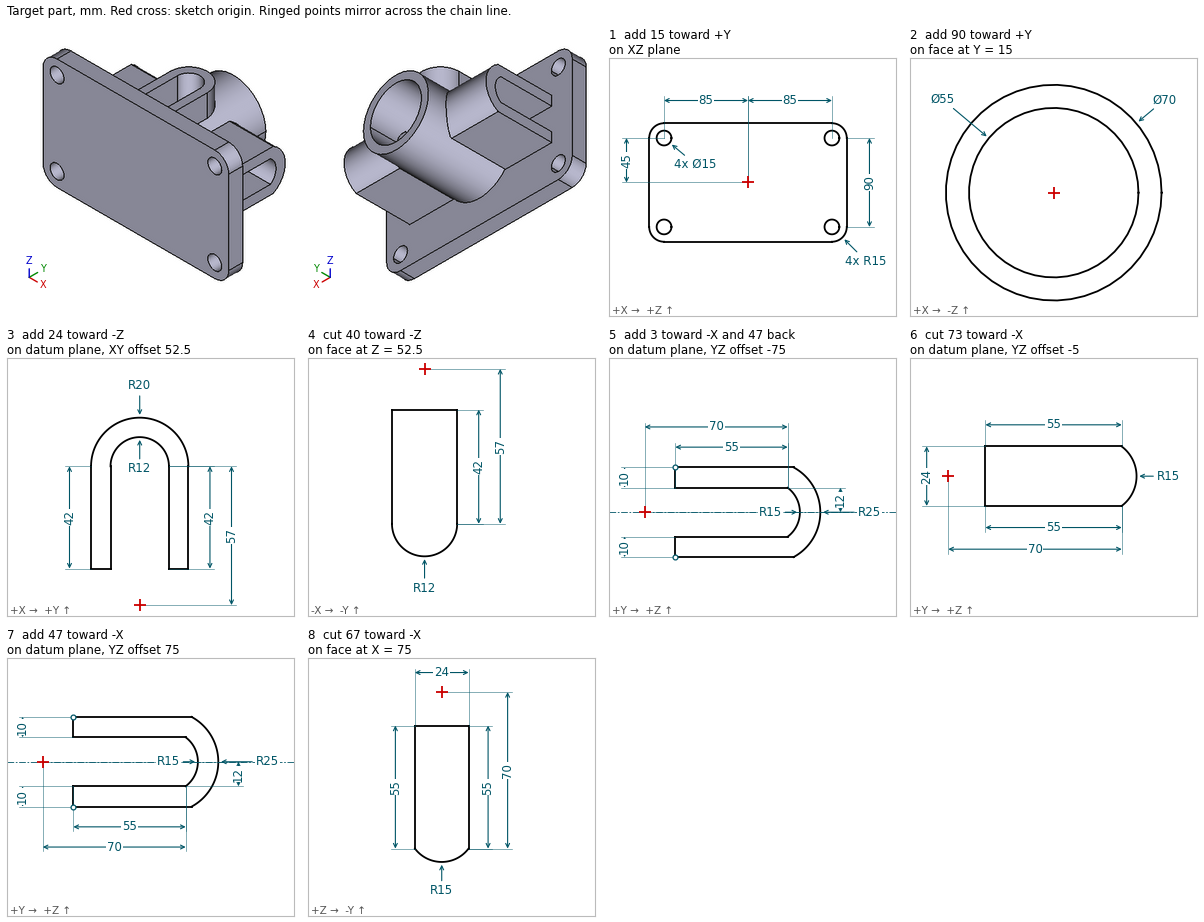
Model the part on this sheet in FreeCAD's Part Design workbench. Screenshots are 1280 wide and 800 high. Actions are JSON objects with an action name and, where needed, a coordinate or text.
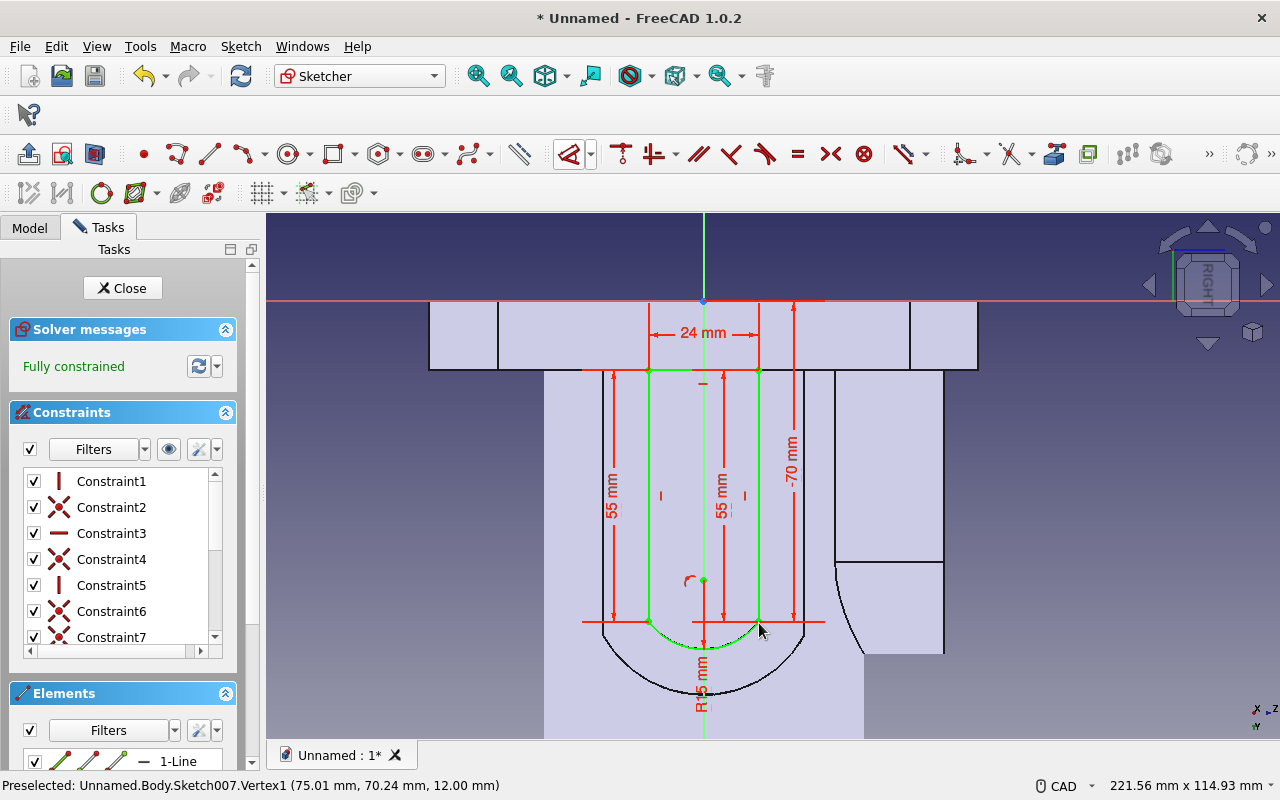
{"action": "left_click", "coordinate": [123, 288]}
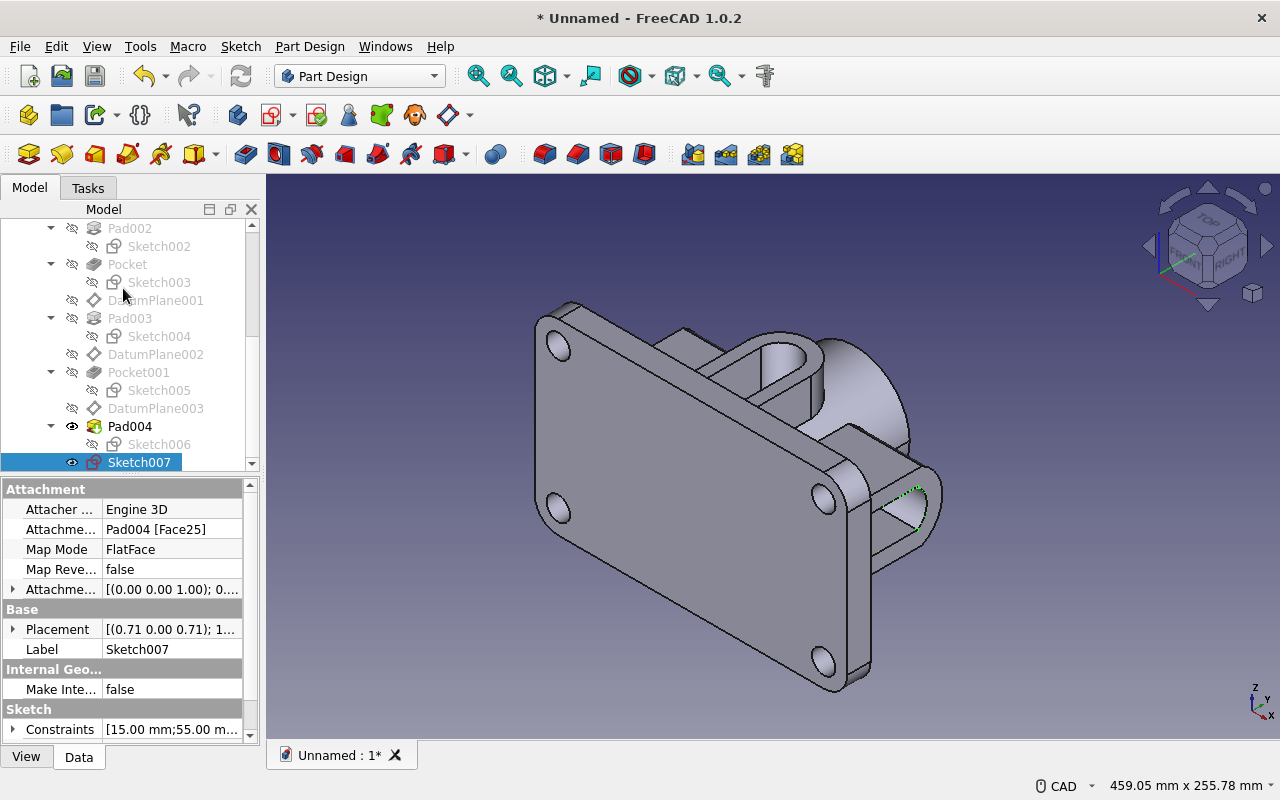
{"action": "left_click", "coordinate": [246, 154]}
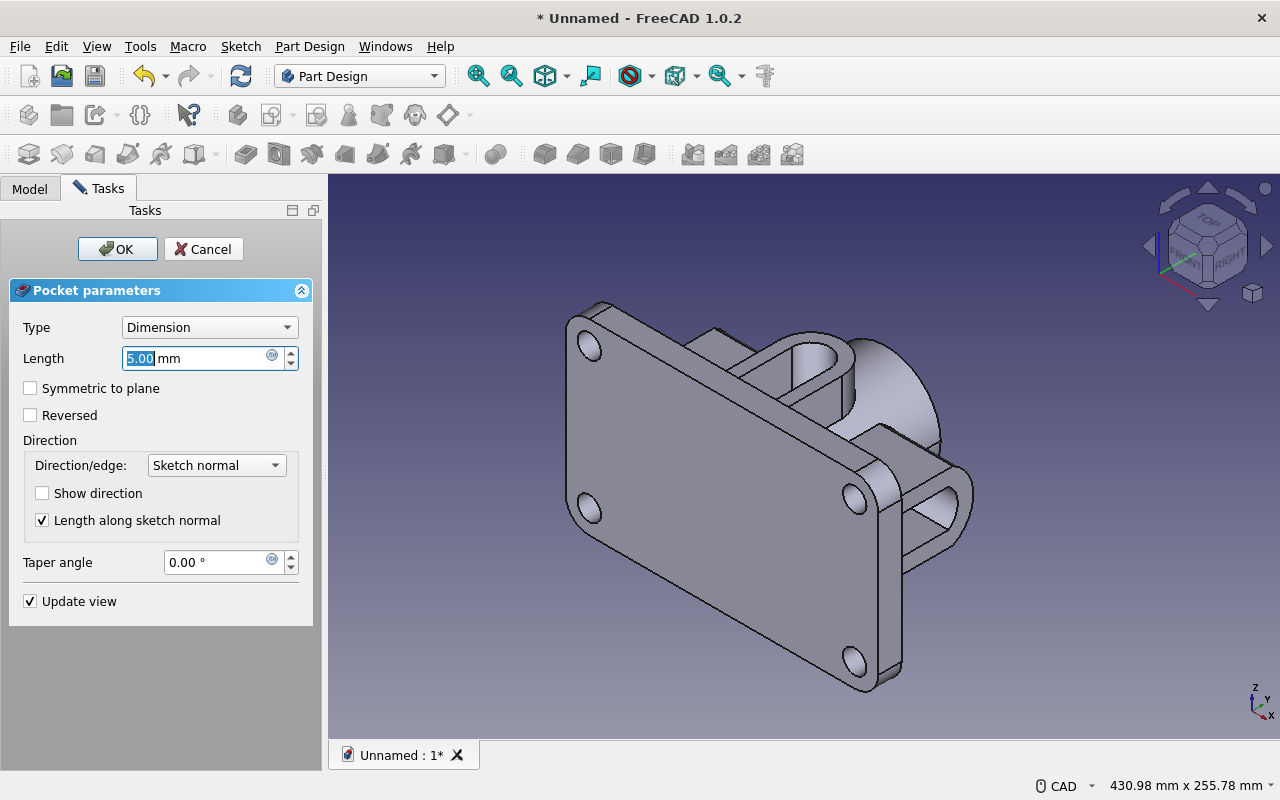
{"action": "type", "text": "67"}
{"action": "key", "text": "Tab"}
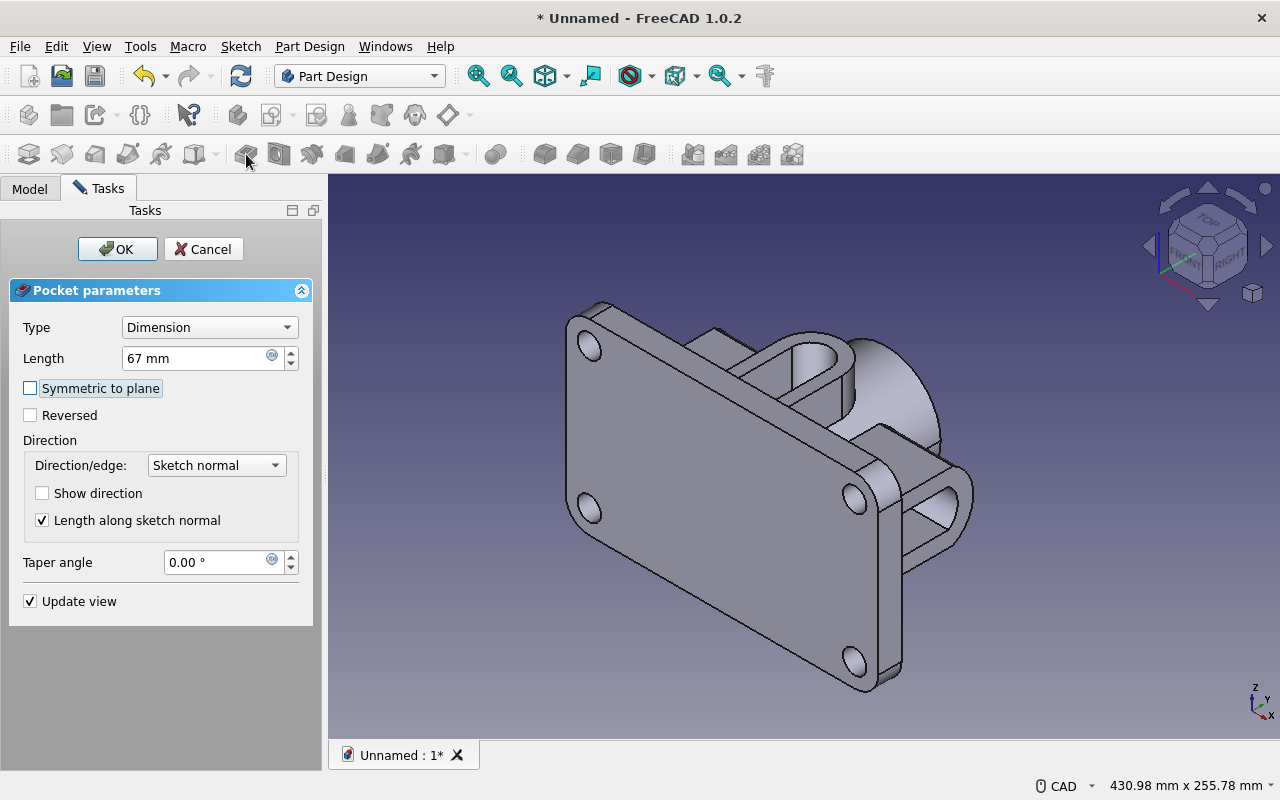
{"action": "left_click", "coordinate": [118, 249]}